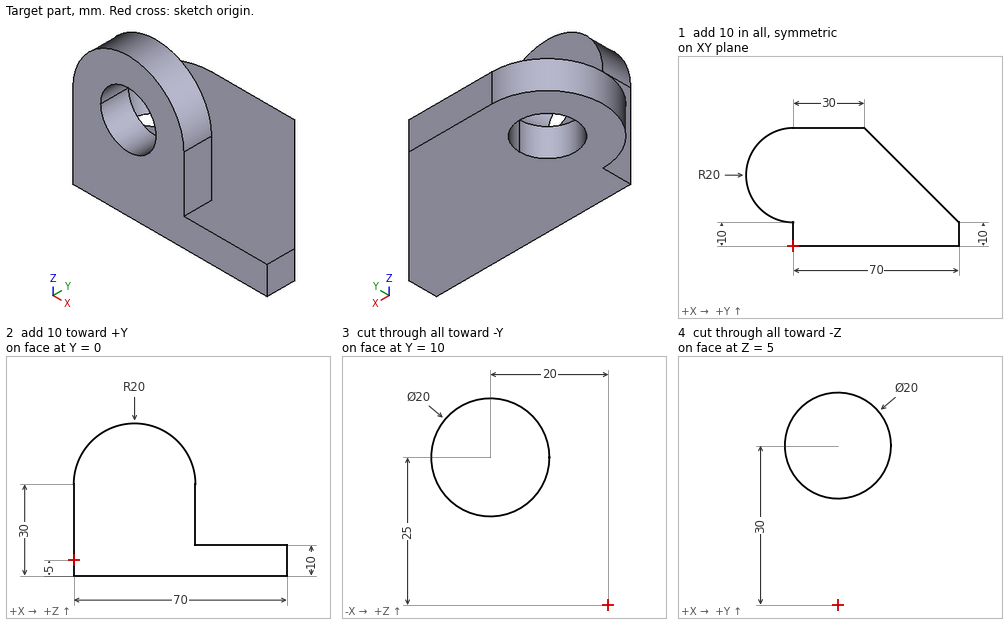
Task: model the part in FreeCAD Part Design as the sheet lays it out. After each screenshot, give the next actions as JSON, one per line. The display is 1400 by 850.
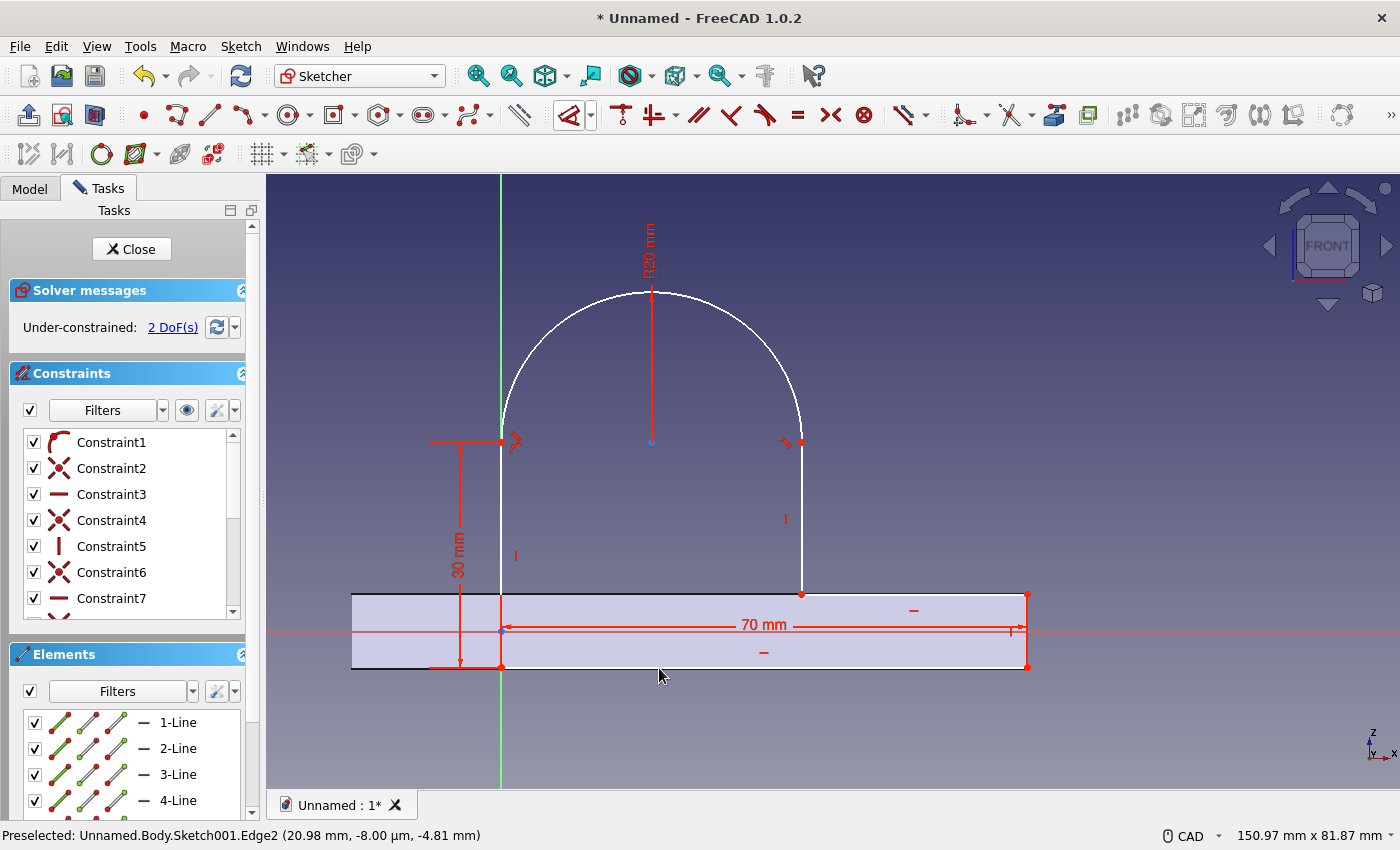
{"action": "left_click", "coordinate": [1027, 646]}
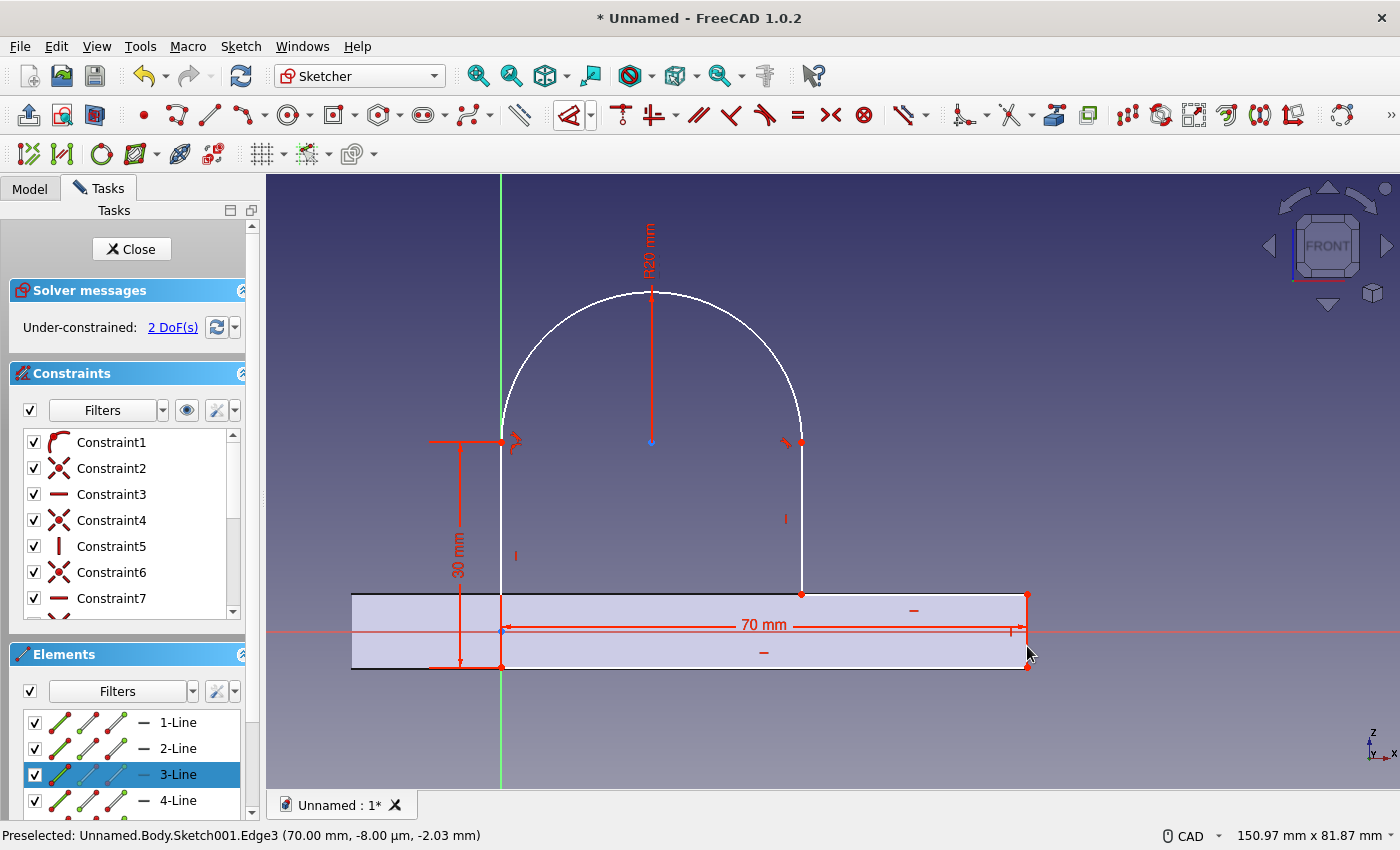
{"action": "left_click", "coordinate": [590, 116]}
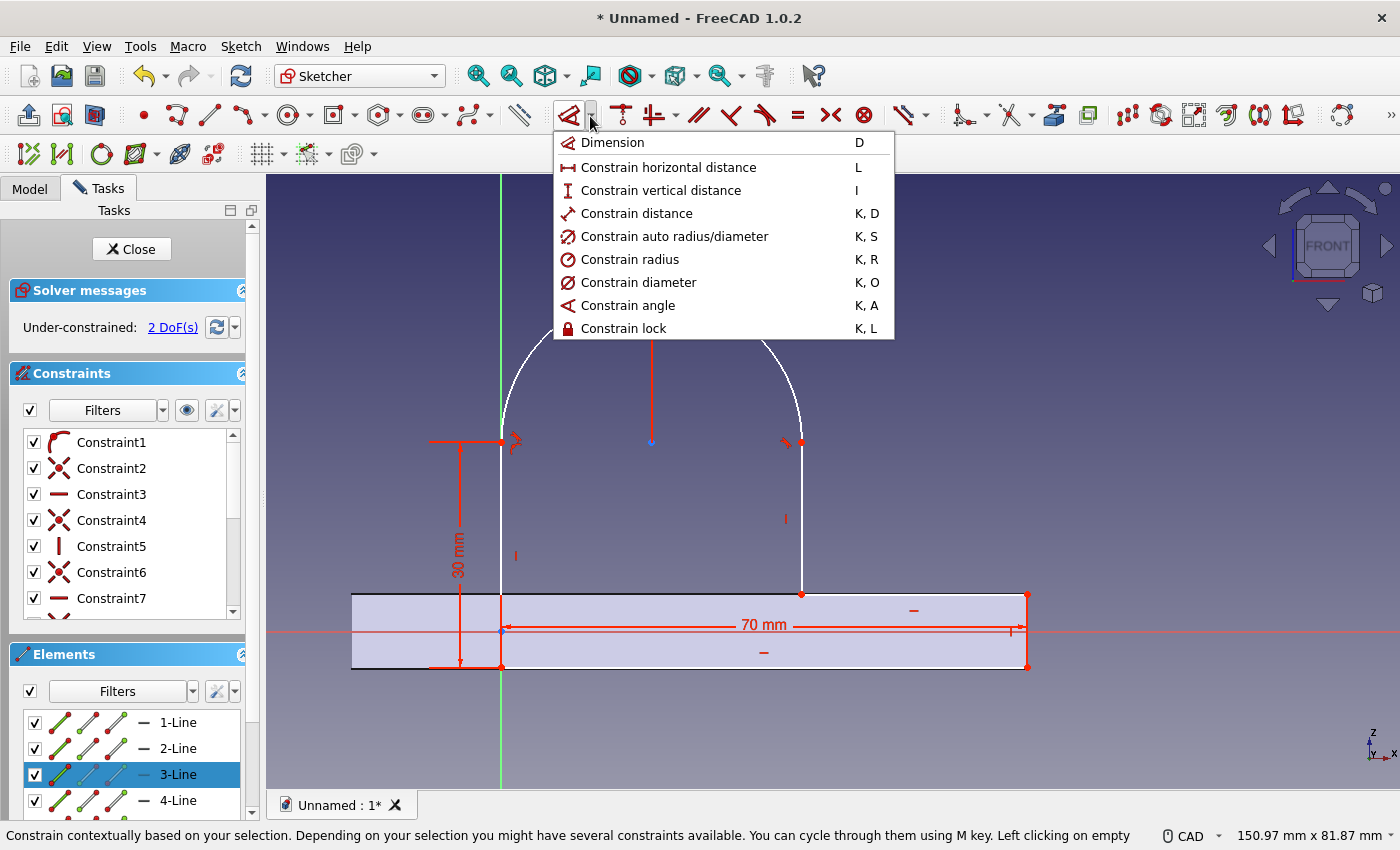
{"action": "left_click", "coordinate": [724, 190]}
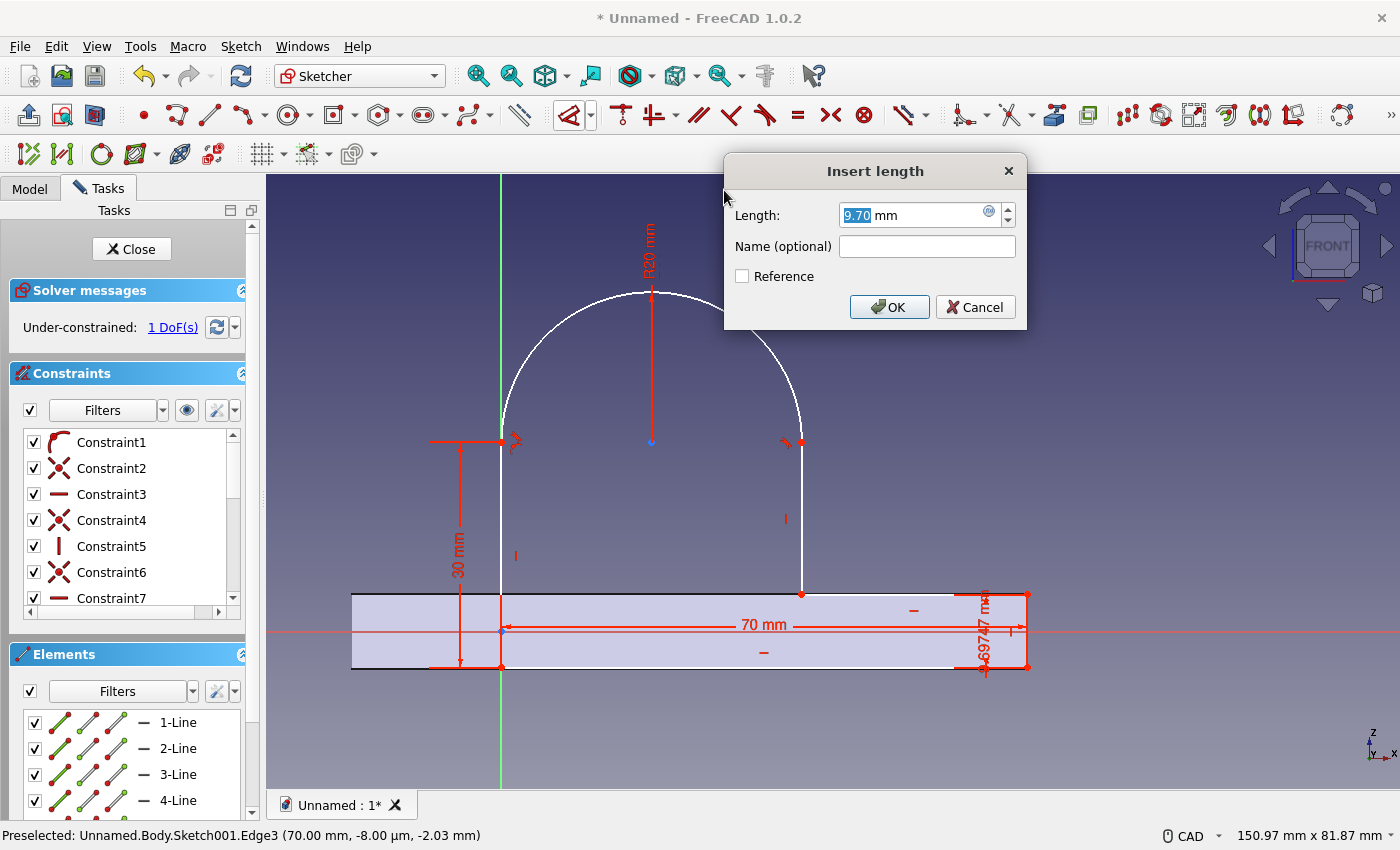
{"action": "type", "text": "10"}
{"action": "key", "text": "Return"}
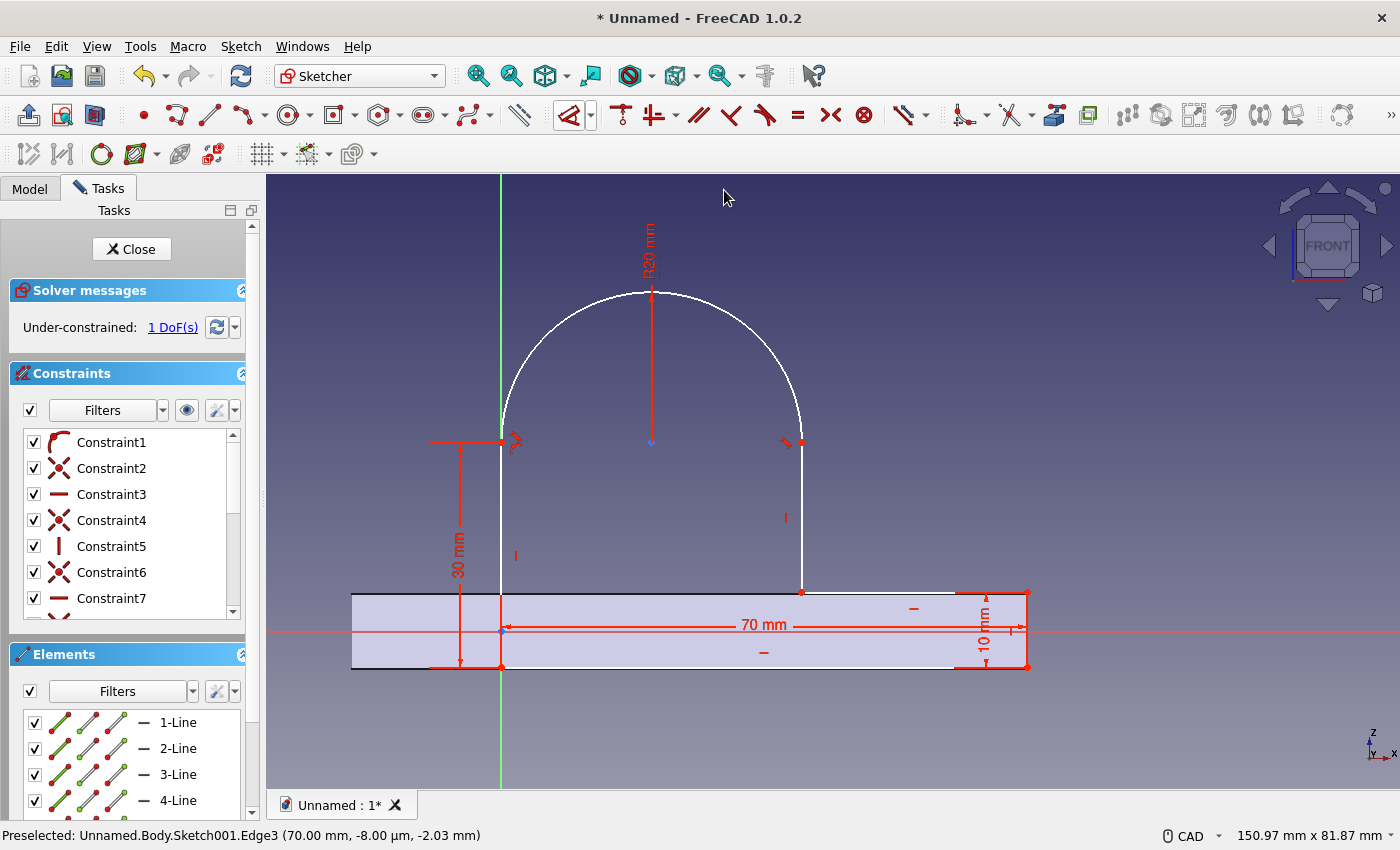
{"action": "left_click", "coordinate": [501, 668]}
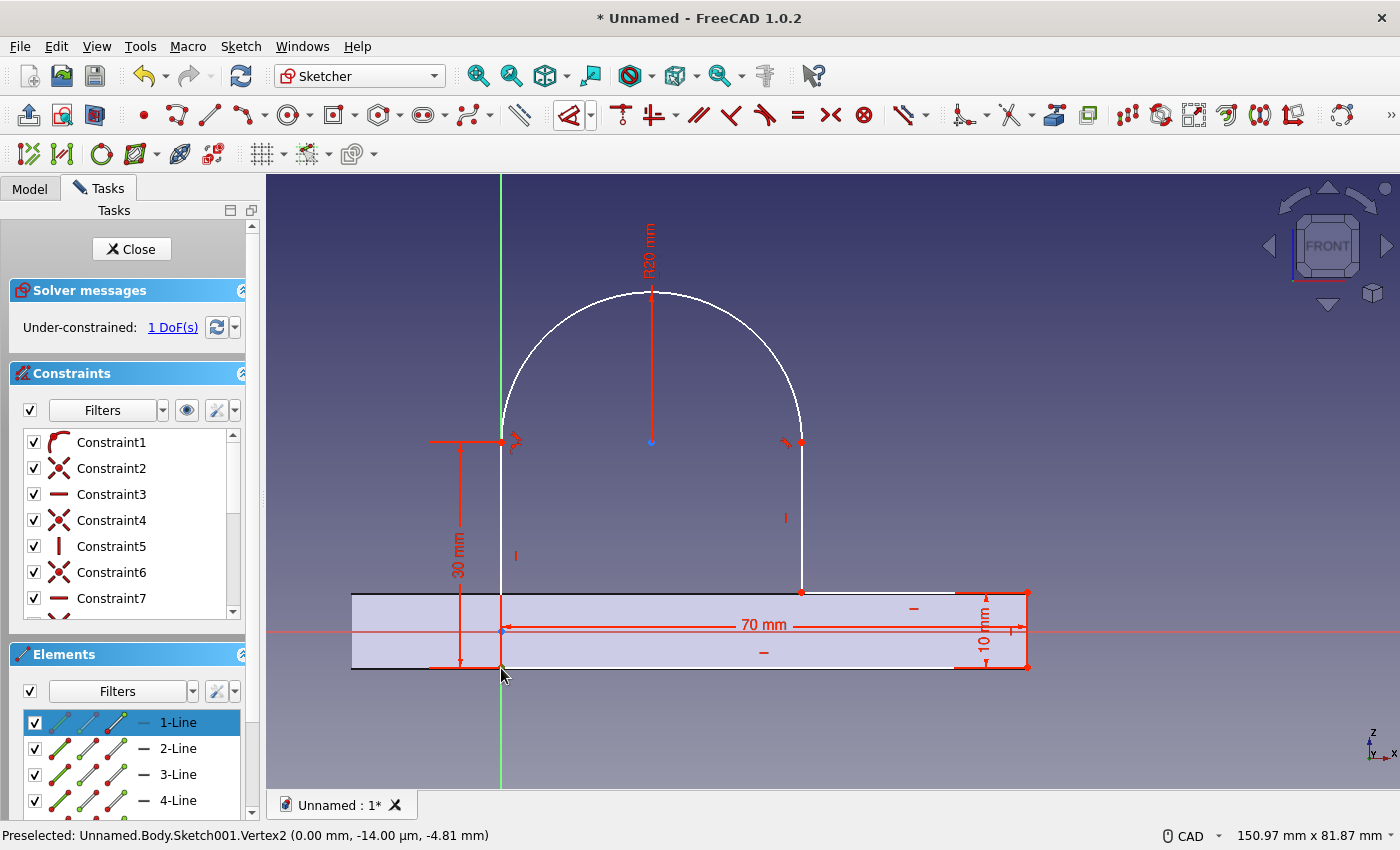
{"action": "left_click", "coordinate": [590, 116]}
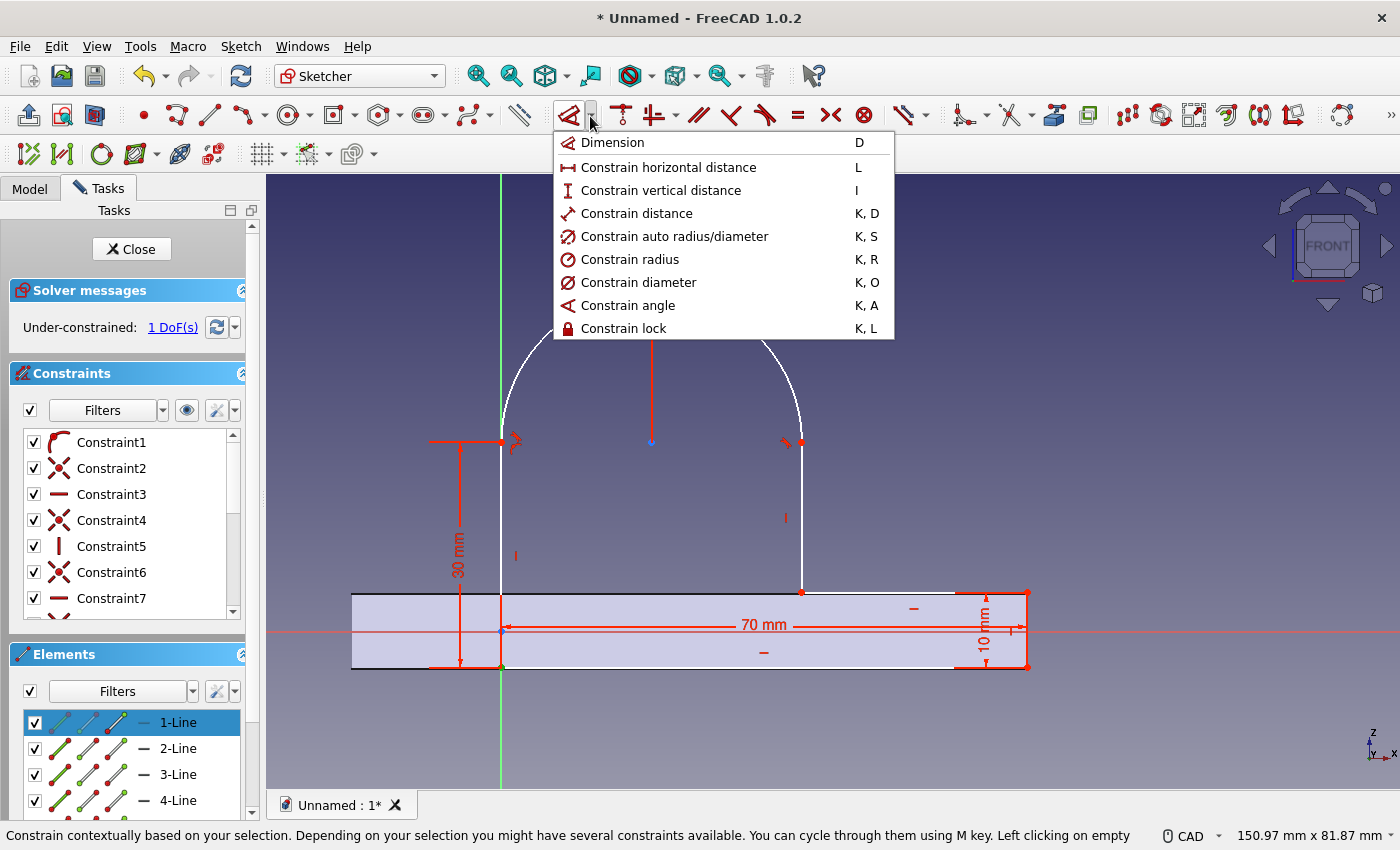
{"action": "left_click", "coordinate": [724, 190]}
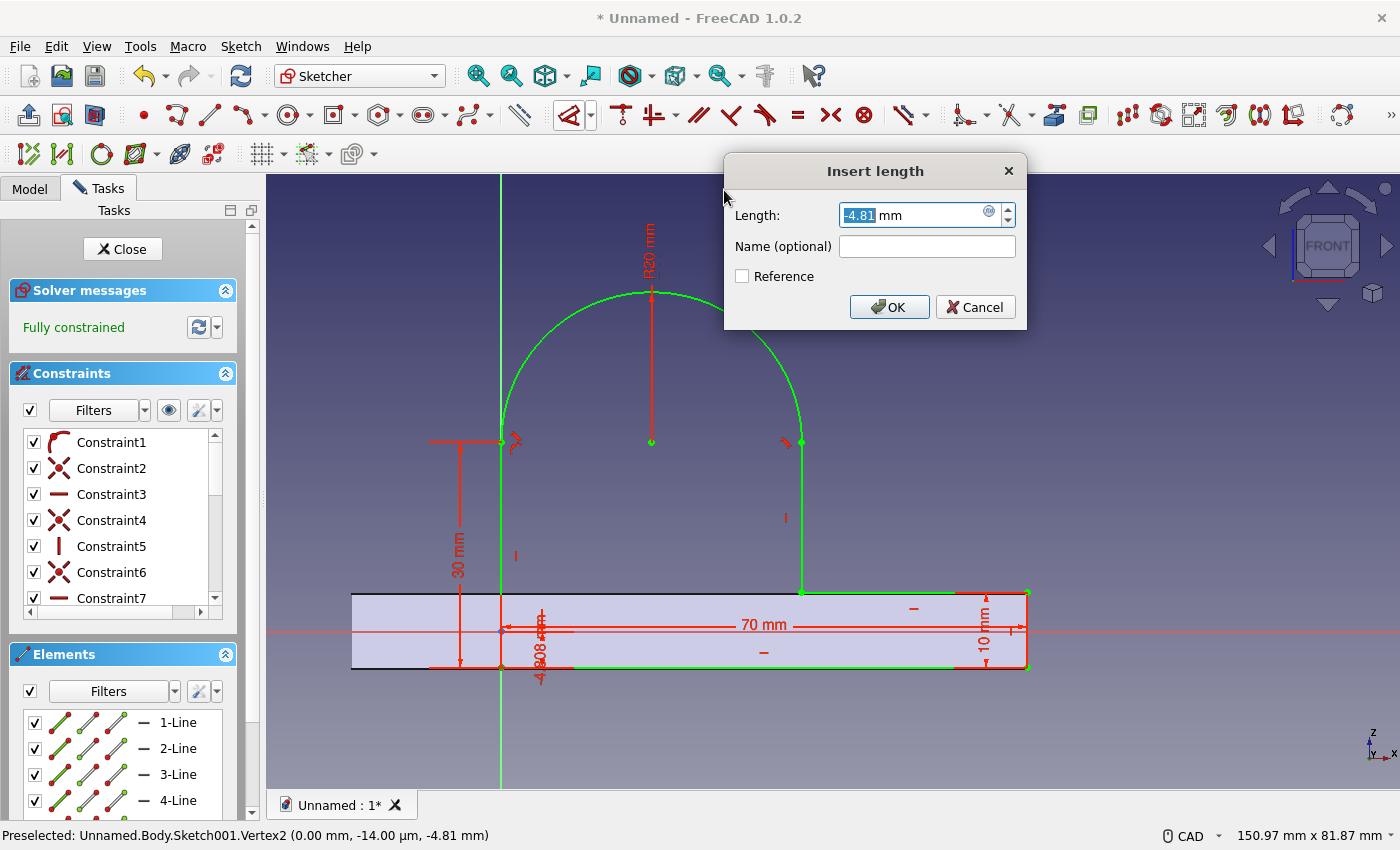
{"action": "type", "text": "-5"}
{"action": "key", "text": "Return"}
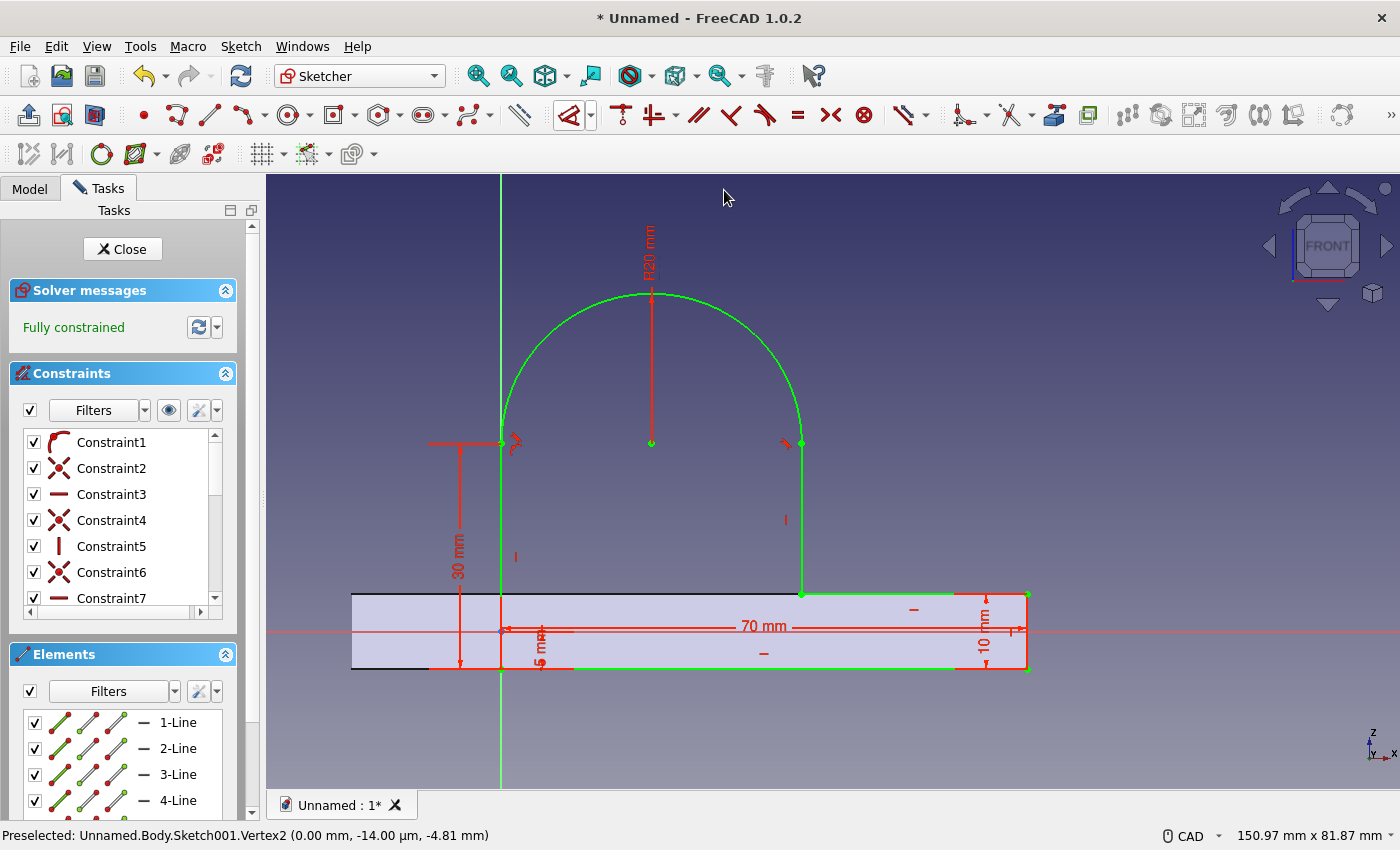
{"action": "left_click", "coordinate": [123, 249]}